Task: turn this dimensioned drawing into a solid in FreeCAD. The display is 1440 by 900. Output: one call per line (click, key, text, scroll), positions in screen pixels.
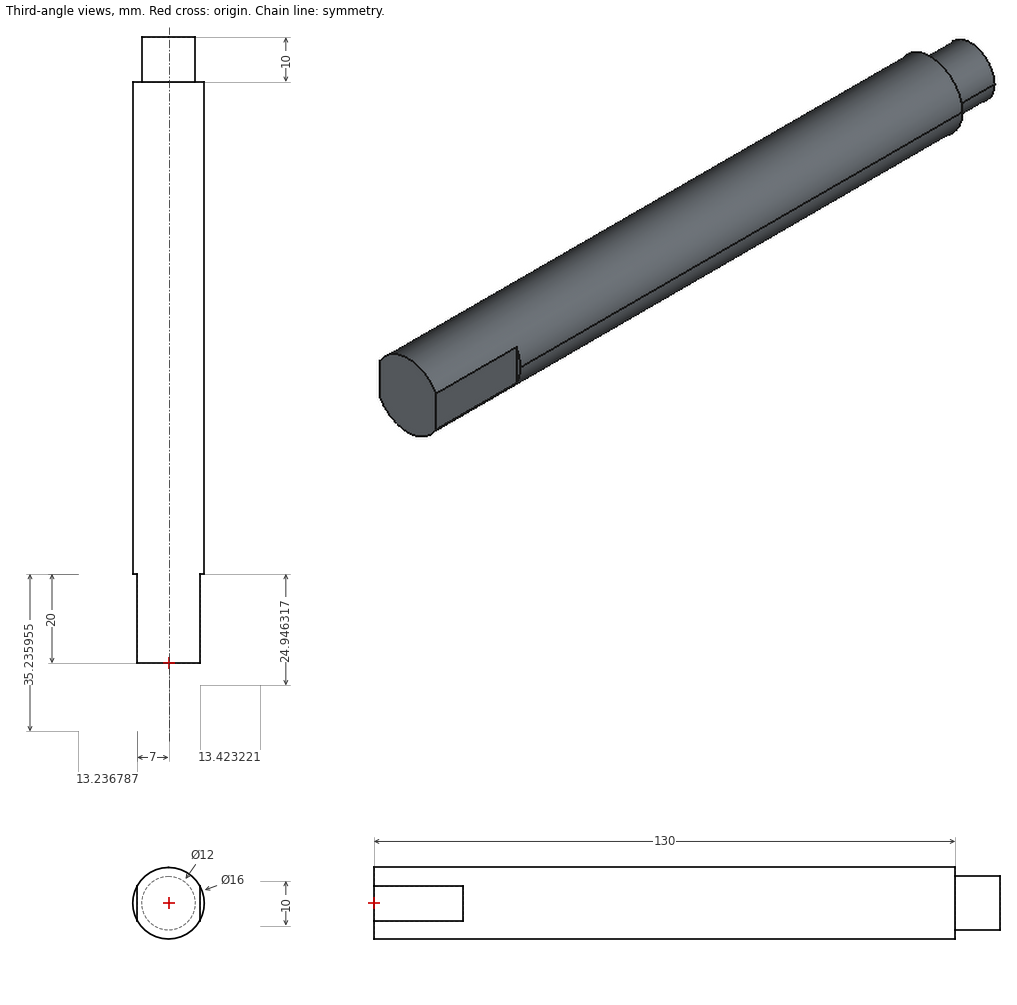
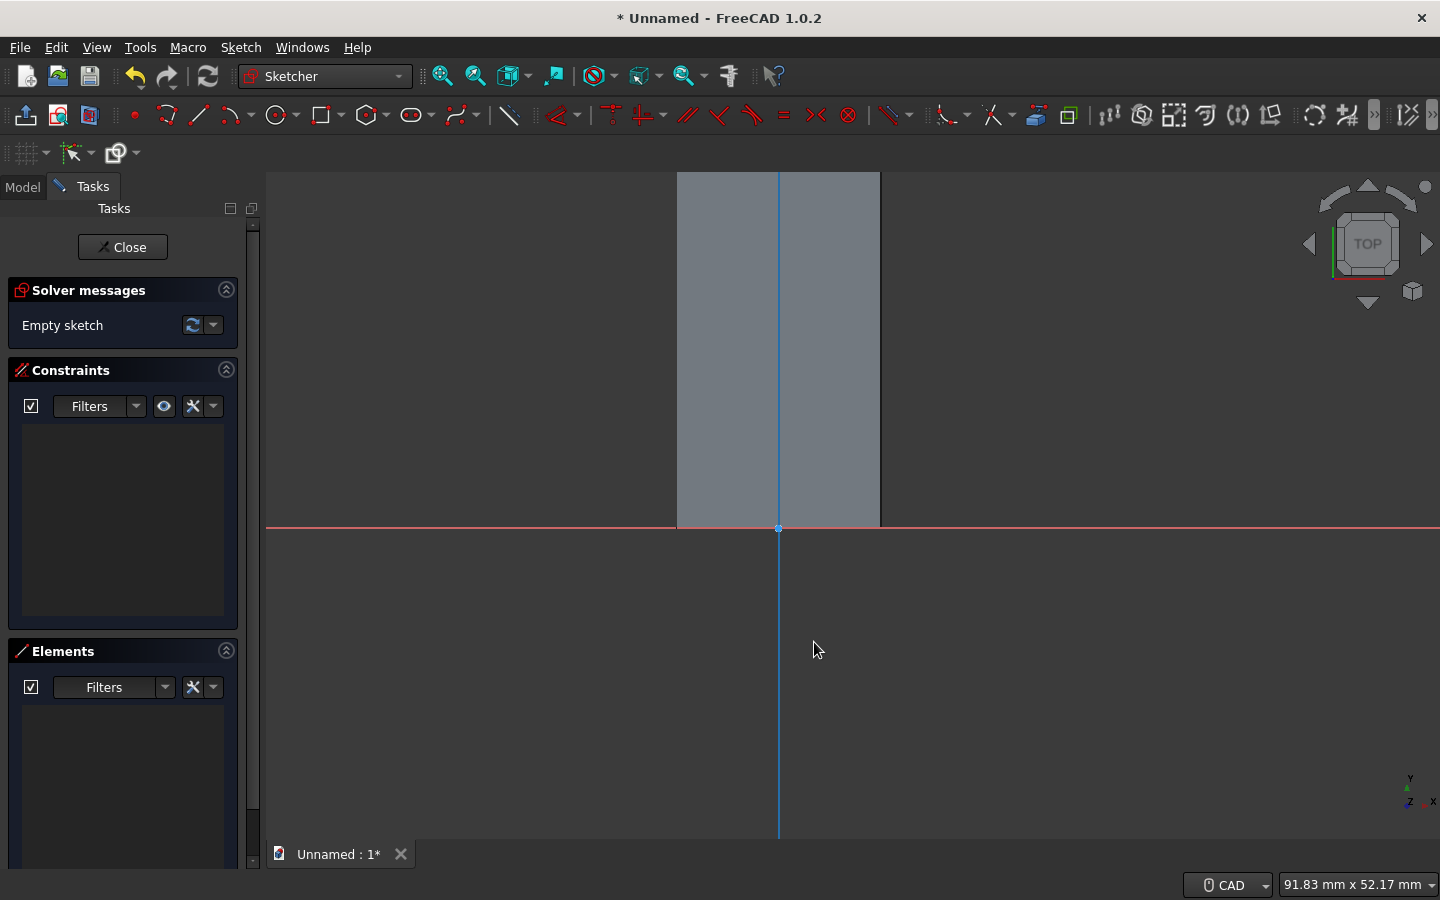
click(322, 116)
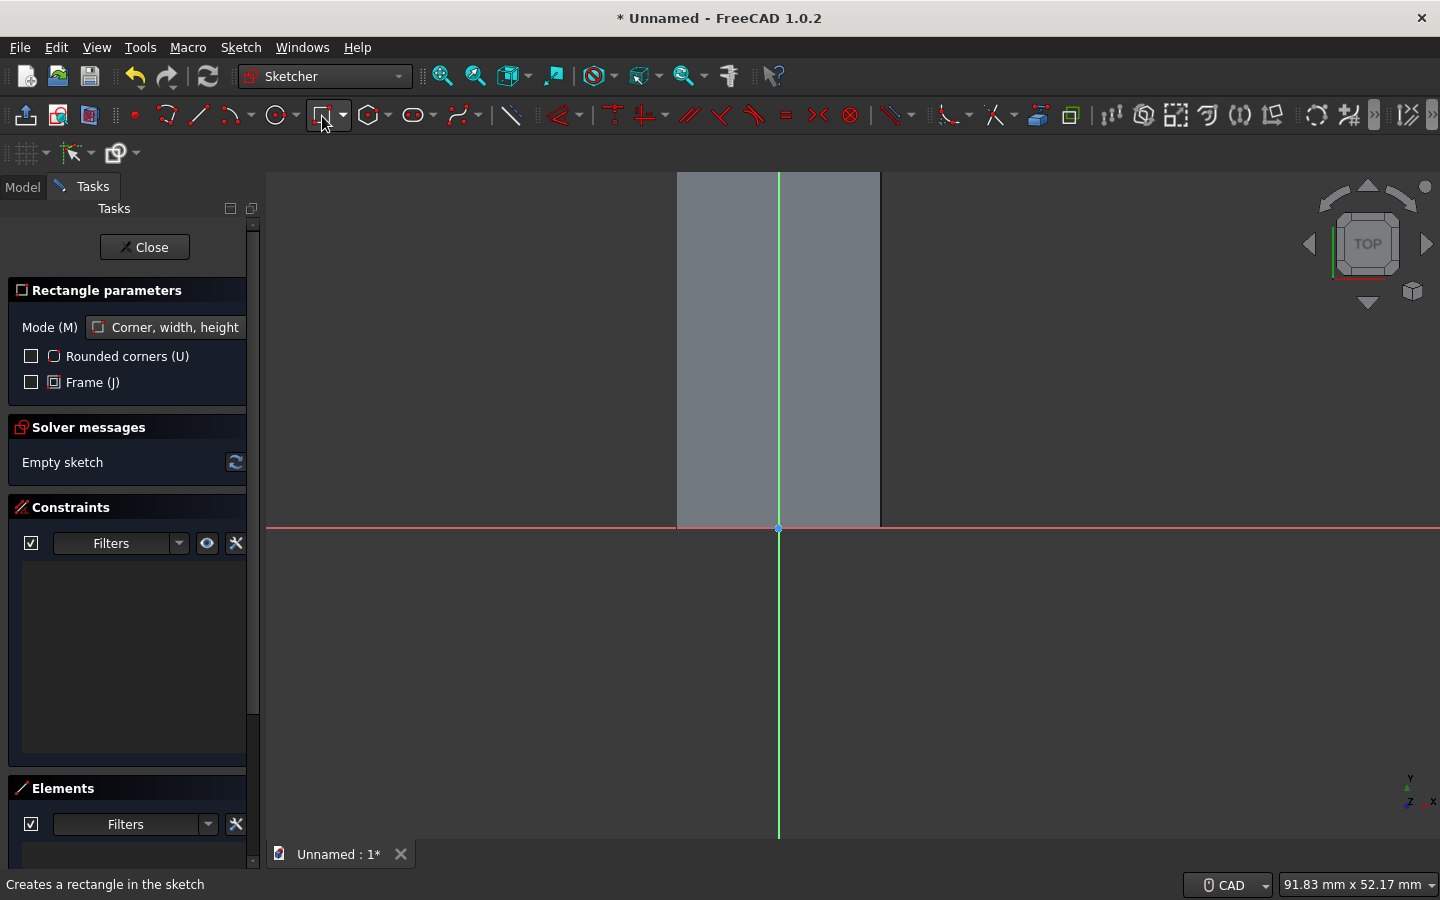
click(520, 273)
click(689, 723)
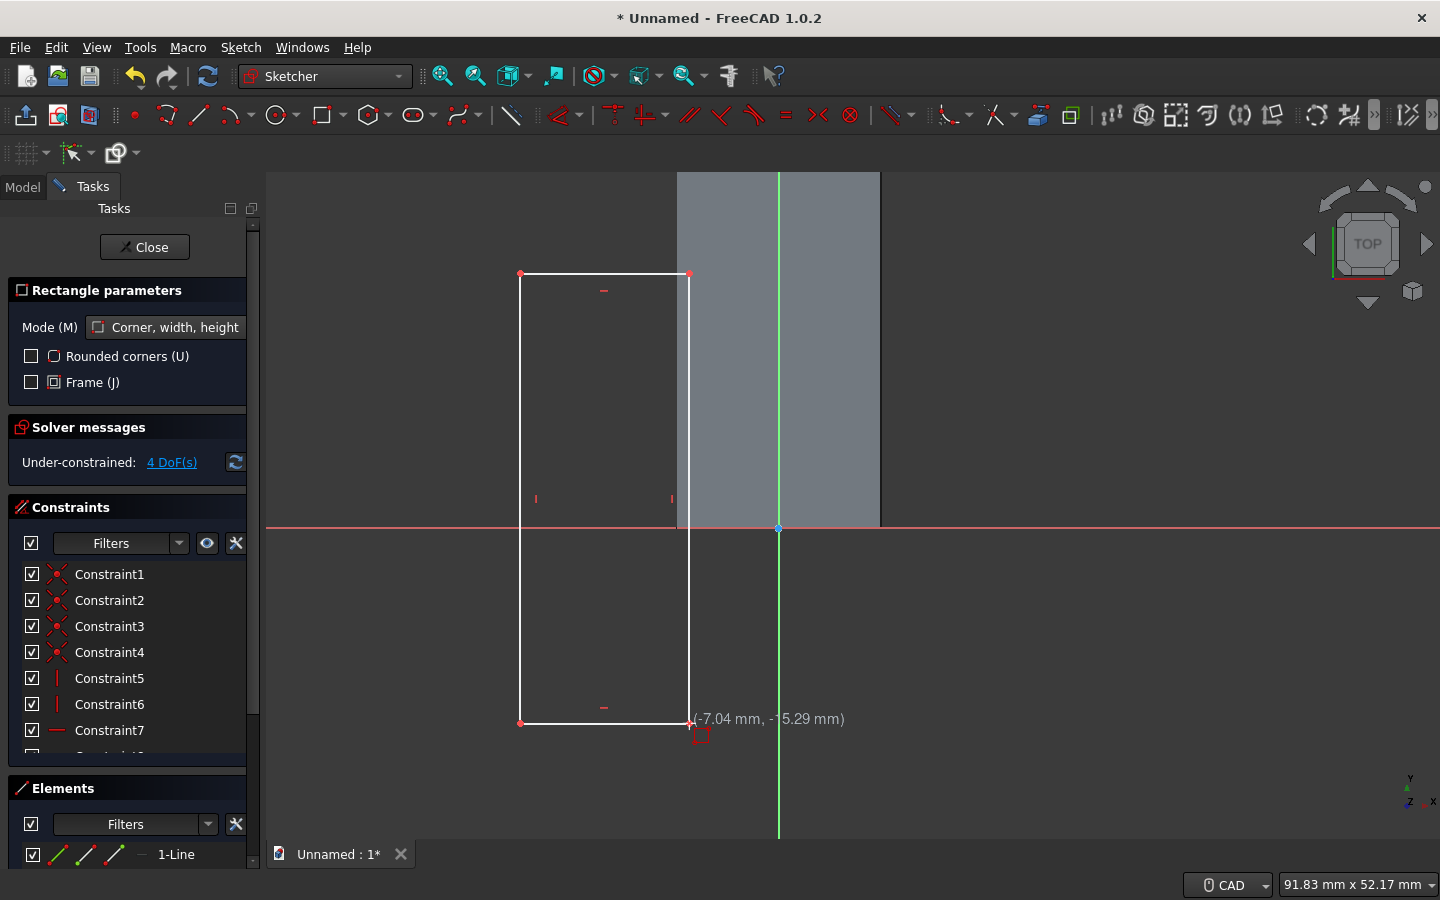
click(868, 273)
click(1040, 592)
key(Escape)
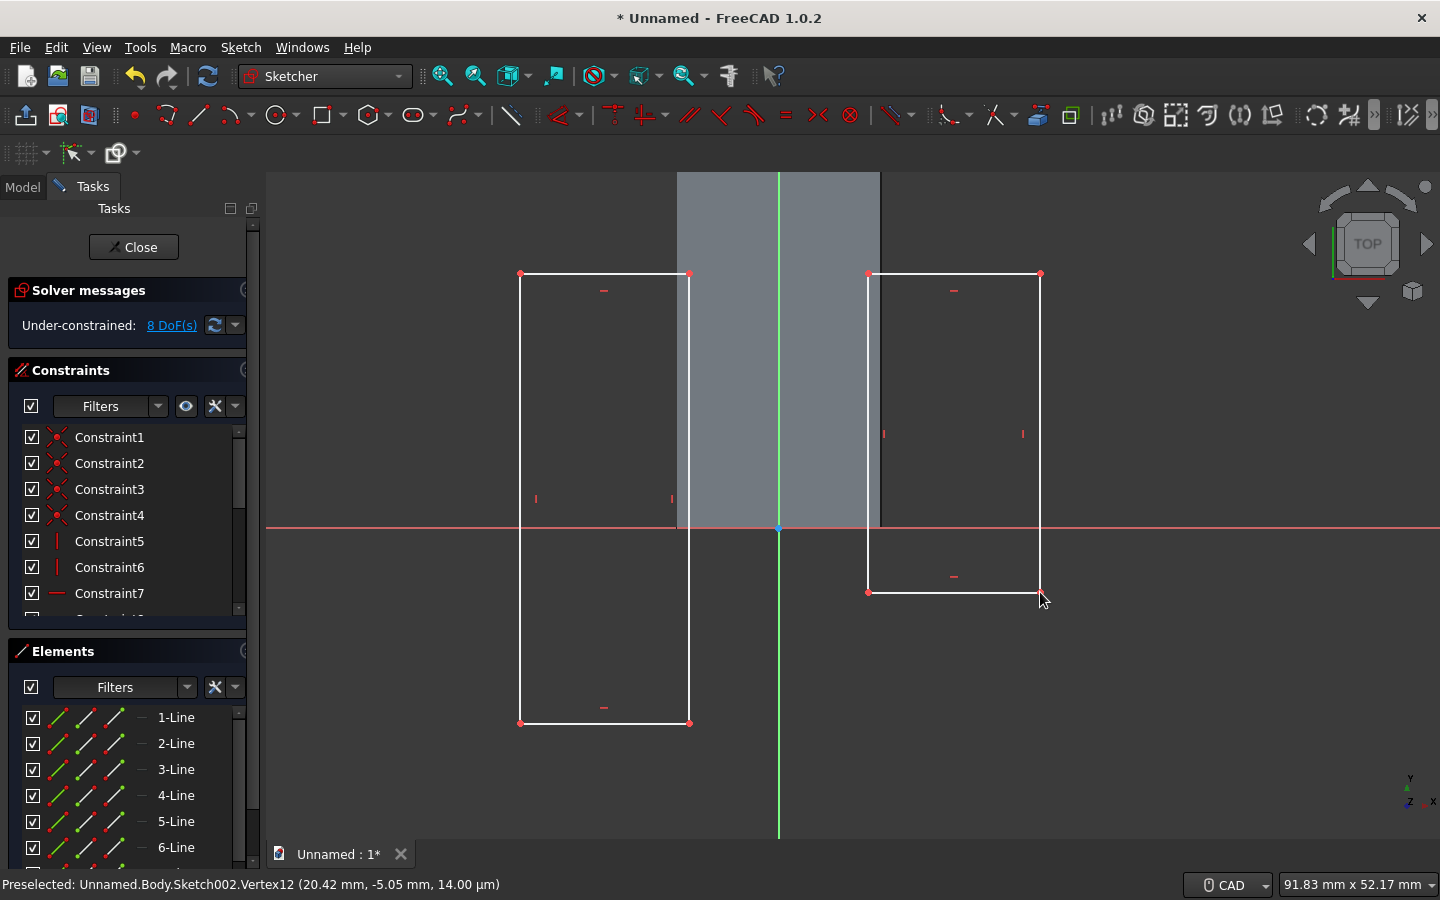
click(689, 274)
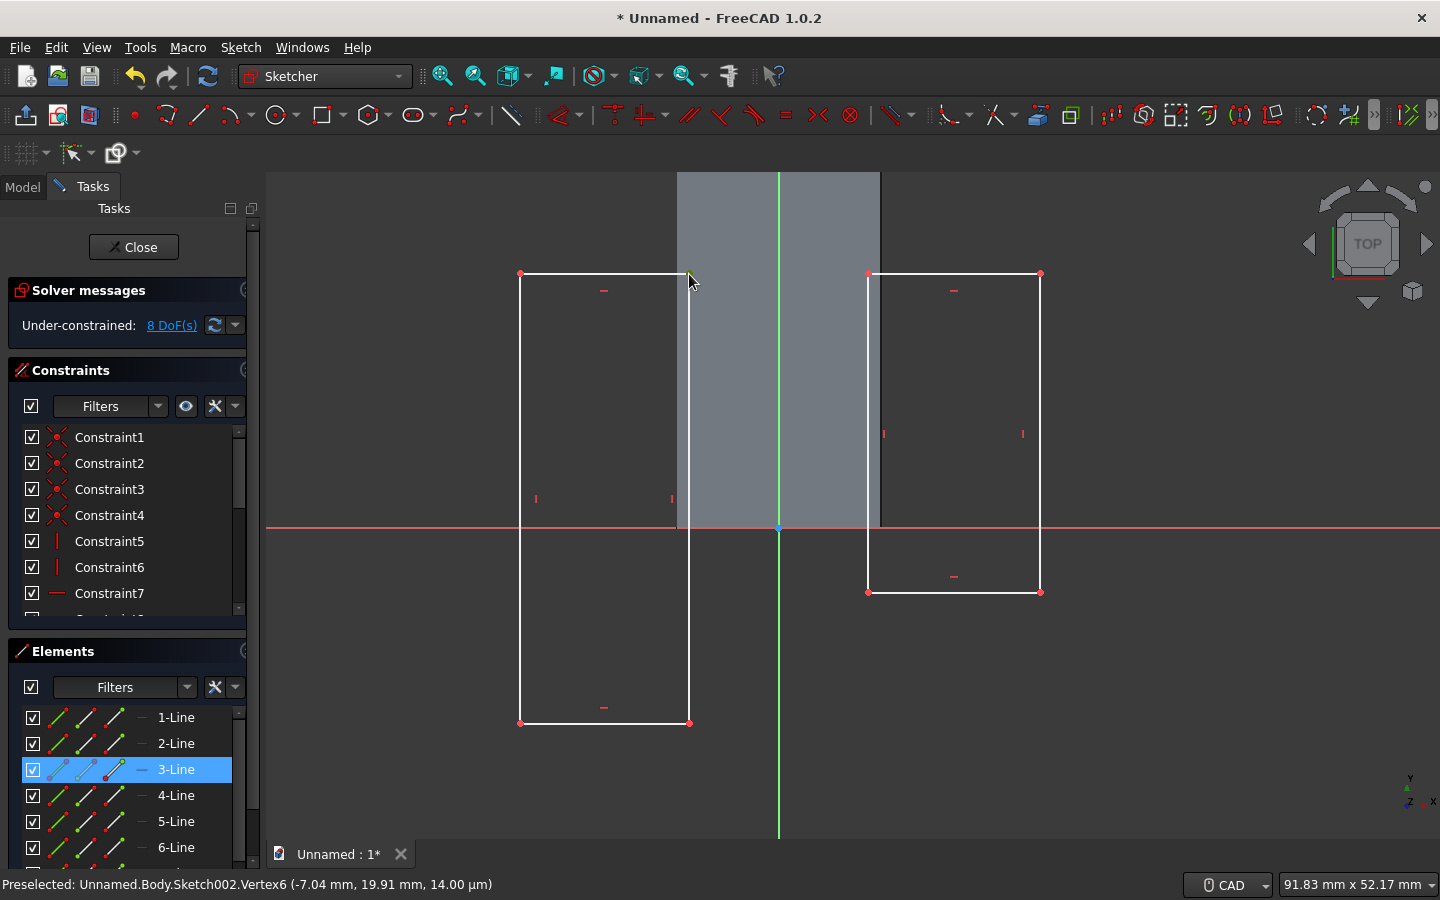
click(868, 274)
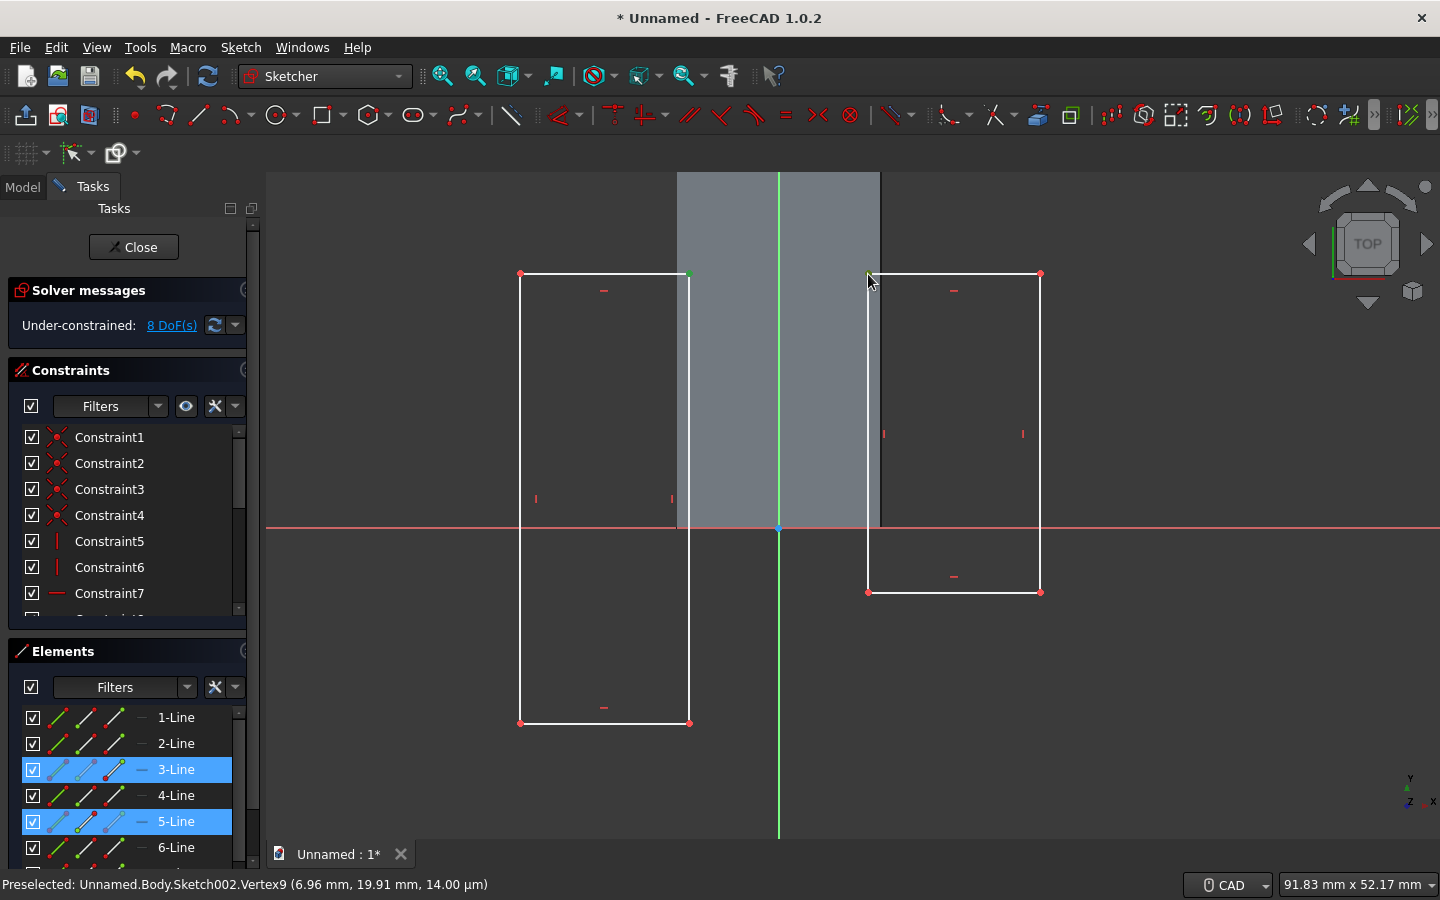
click(779, 767)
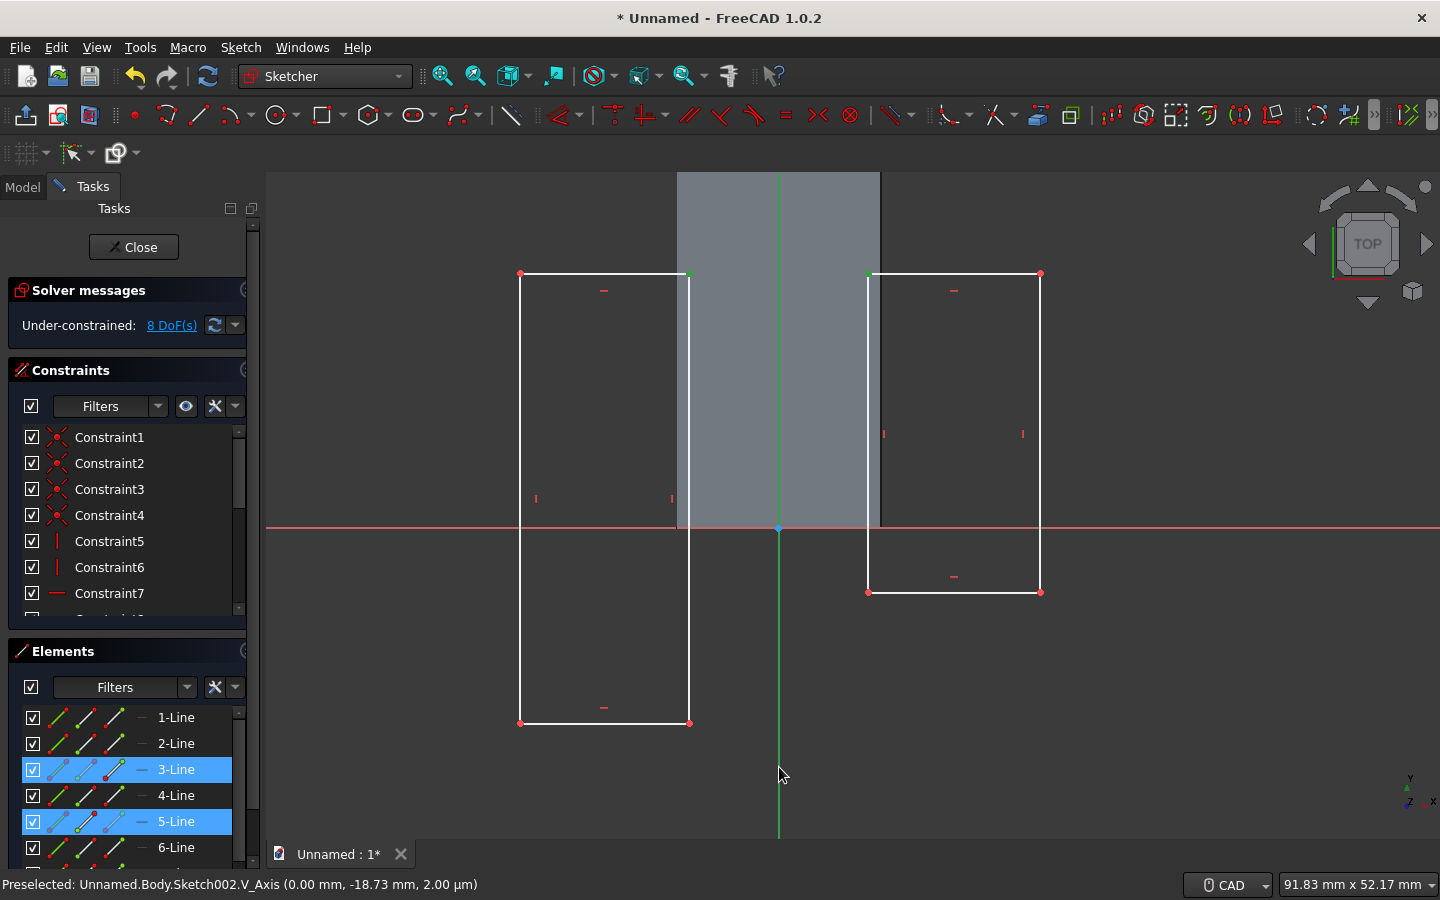
key(s)